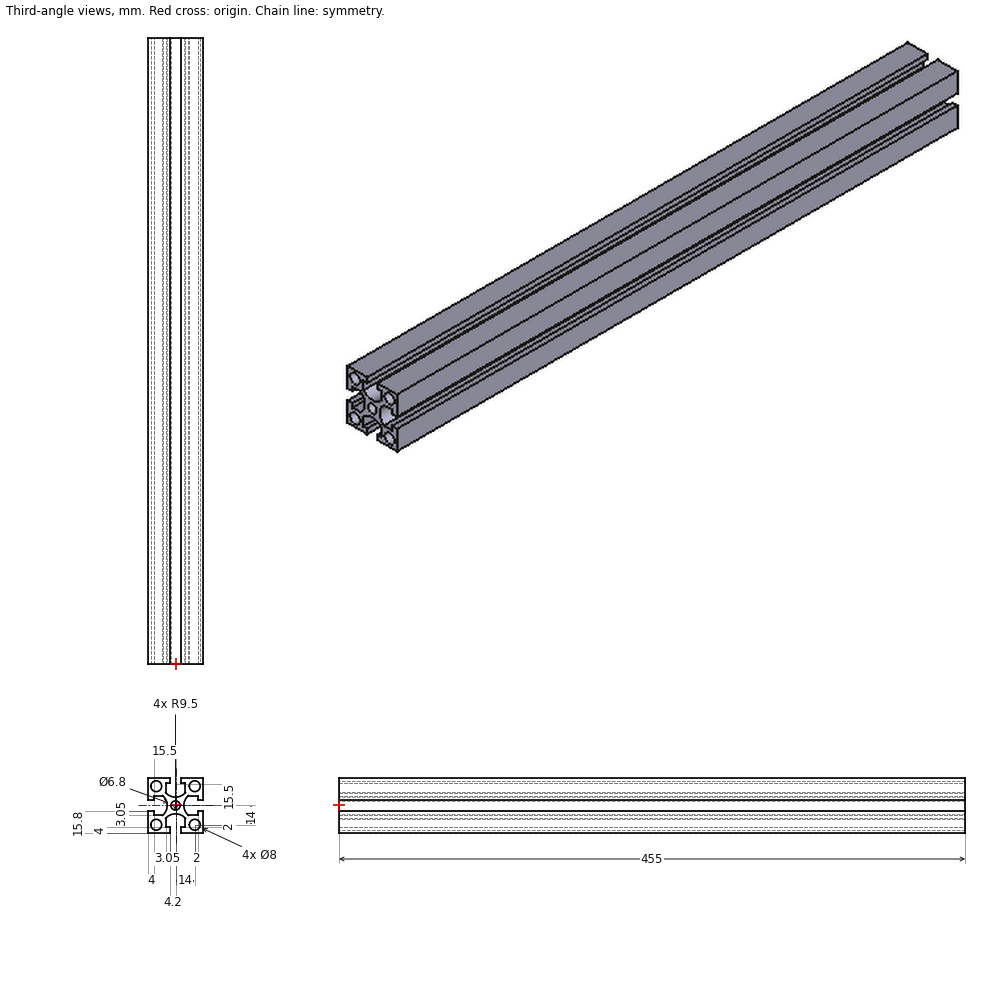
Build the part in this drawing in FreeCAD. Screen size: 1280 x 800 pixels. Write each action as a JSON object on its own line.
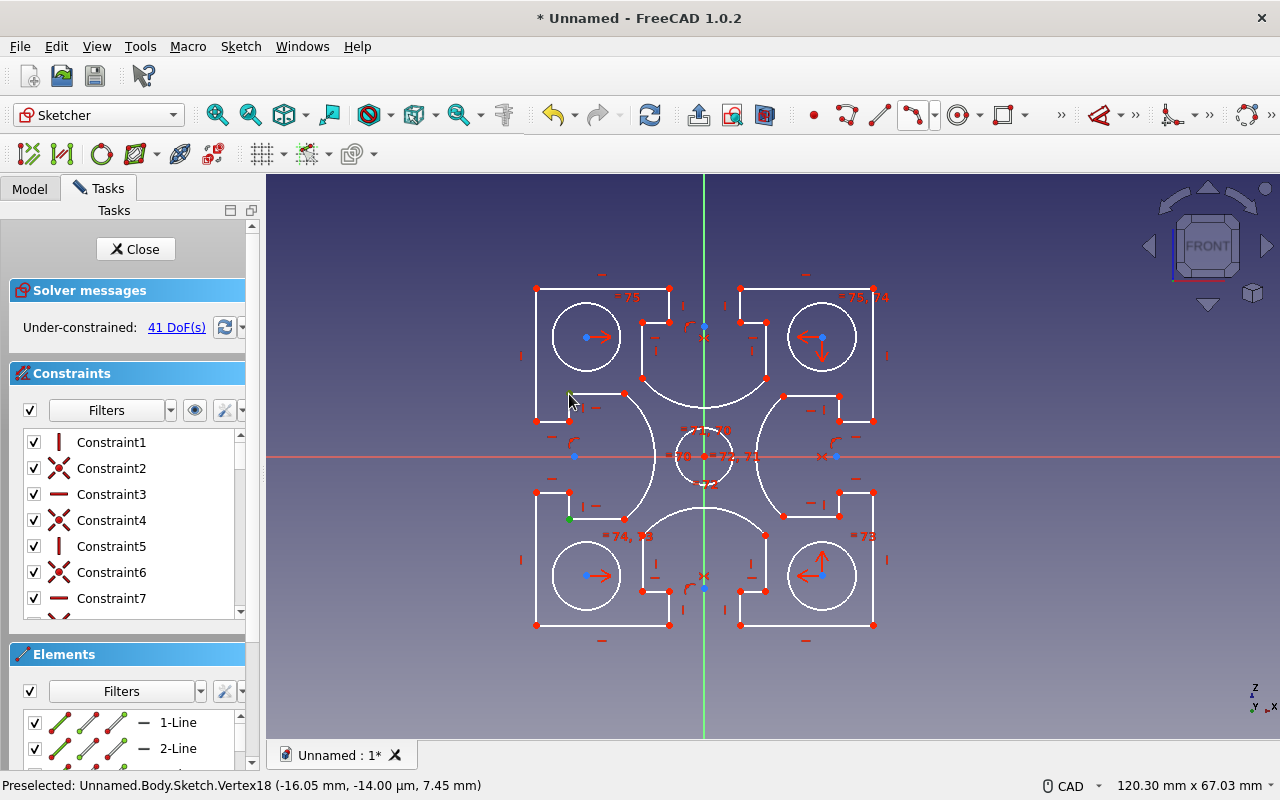
{"action": "left_click", "coordinate": [353, 456]}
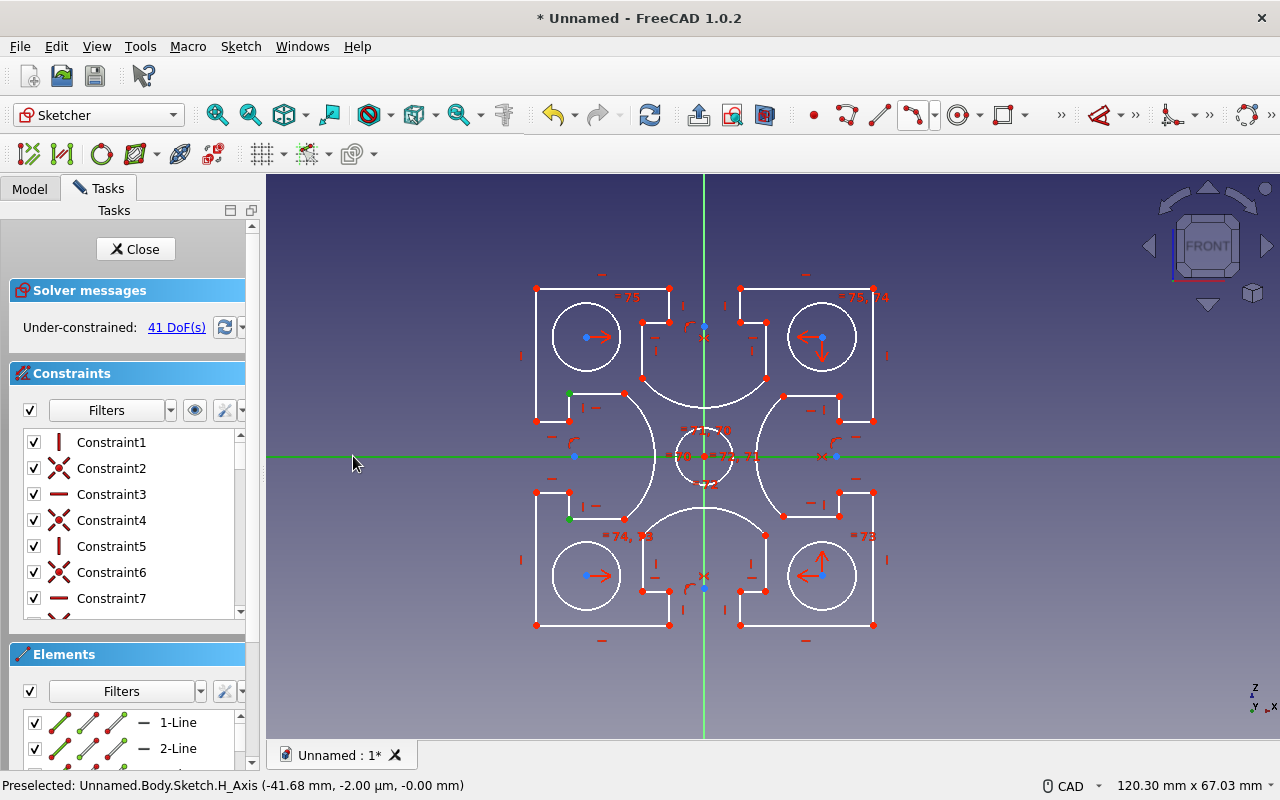
{"action": "key", "text": "s"}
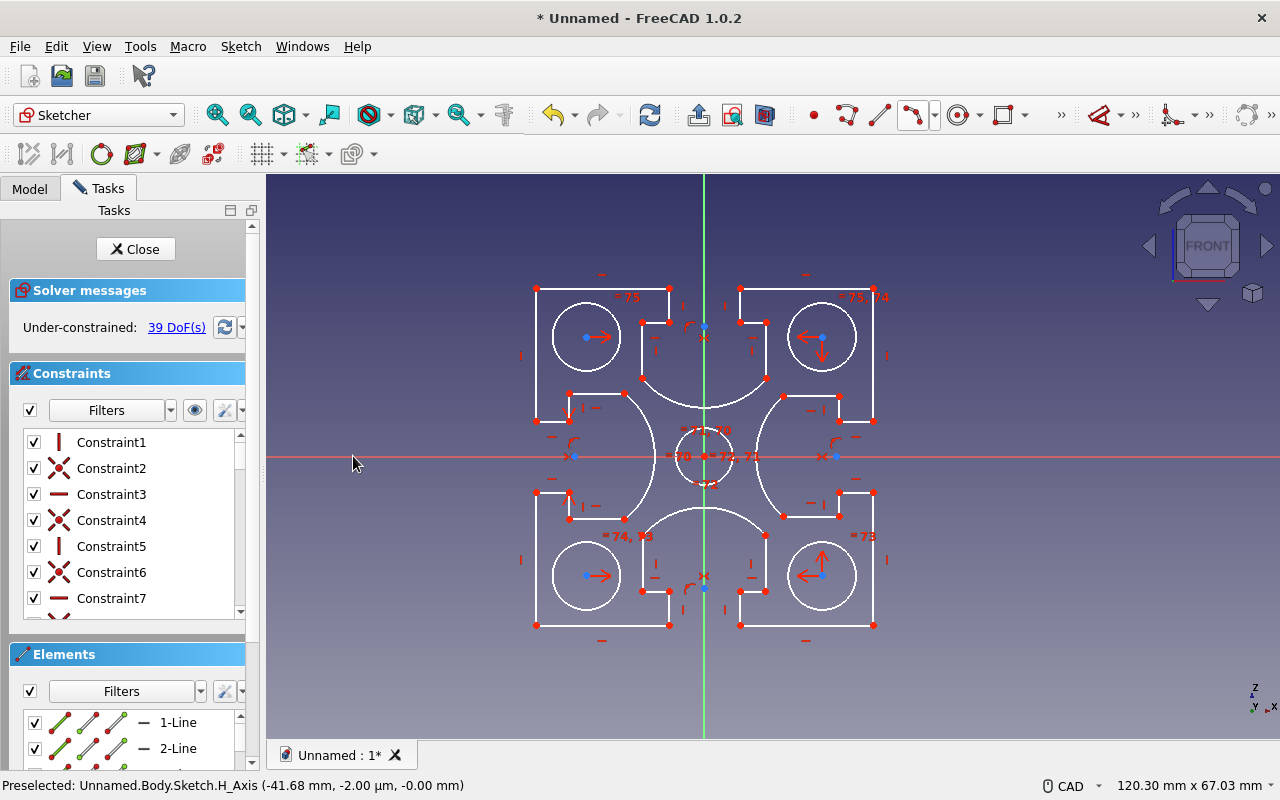
{"action": "left_click", "coordinate": [536, 493]}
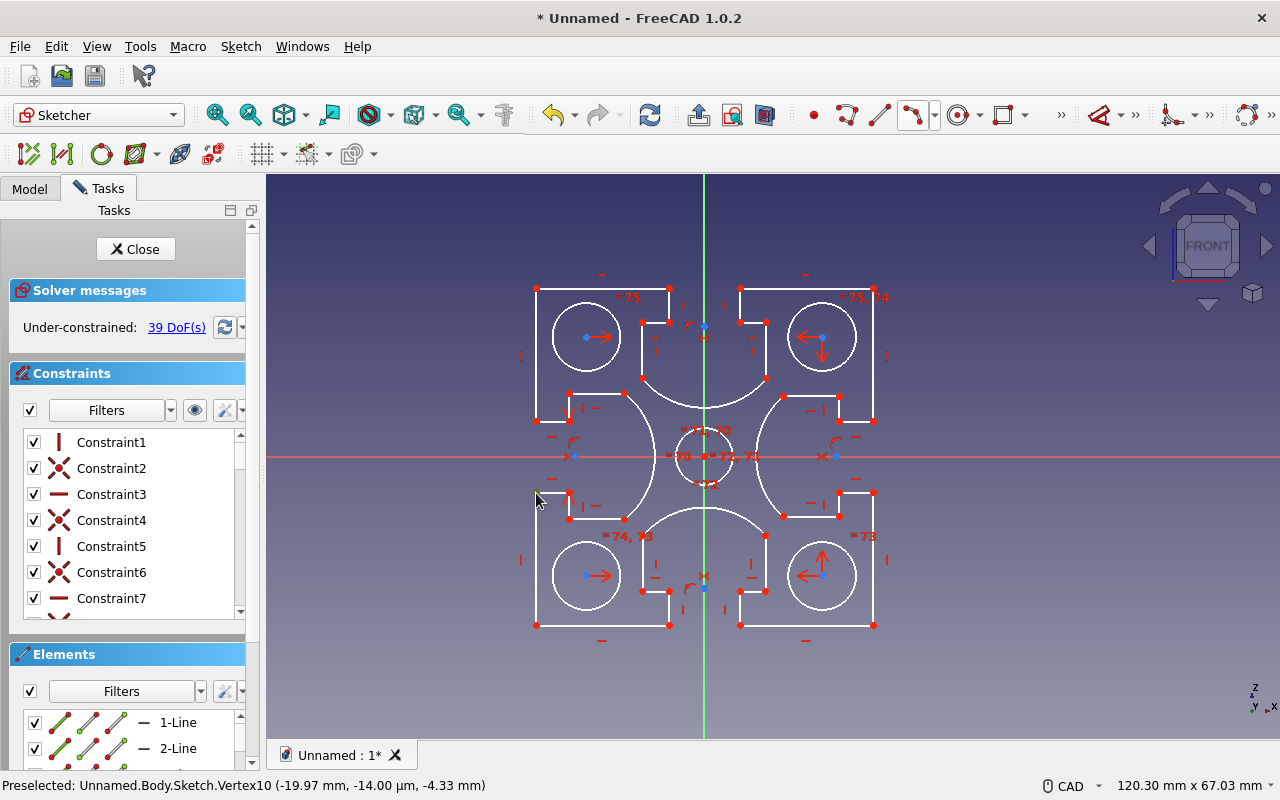
{"action": "left_click", "coordinate": [536, 422]}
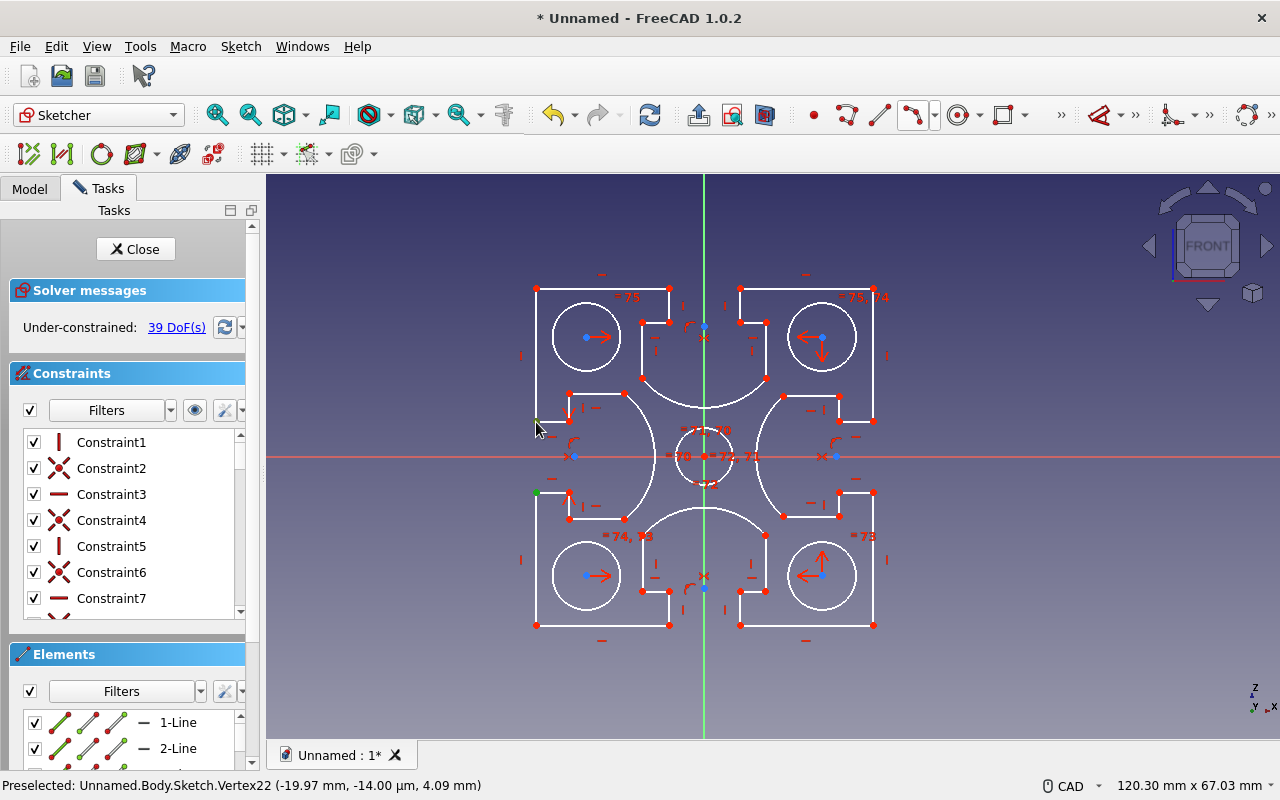
{"action": "left_click", "coordinate": [353, 456]}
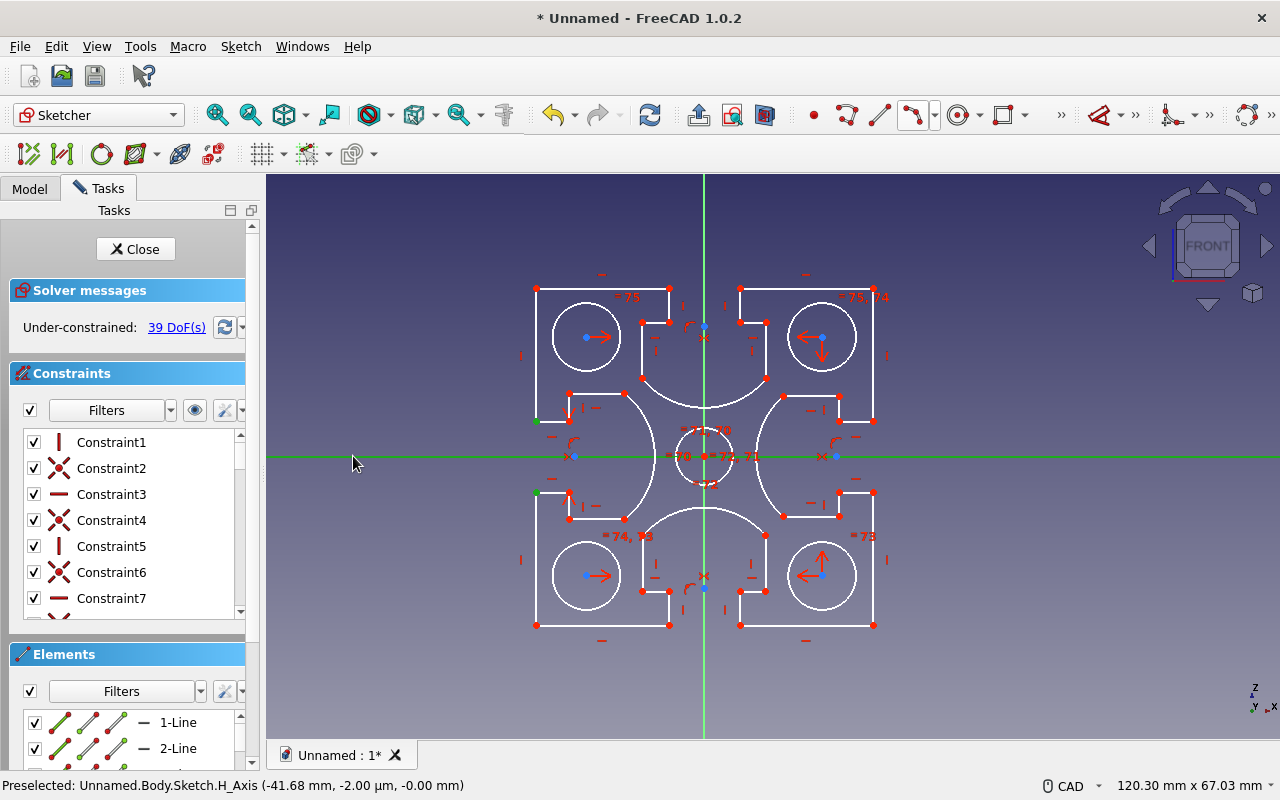
{"action": "key", "text": "s"}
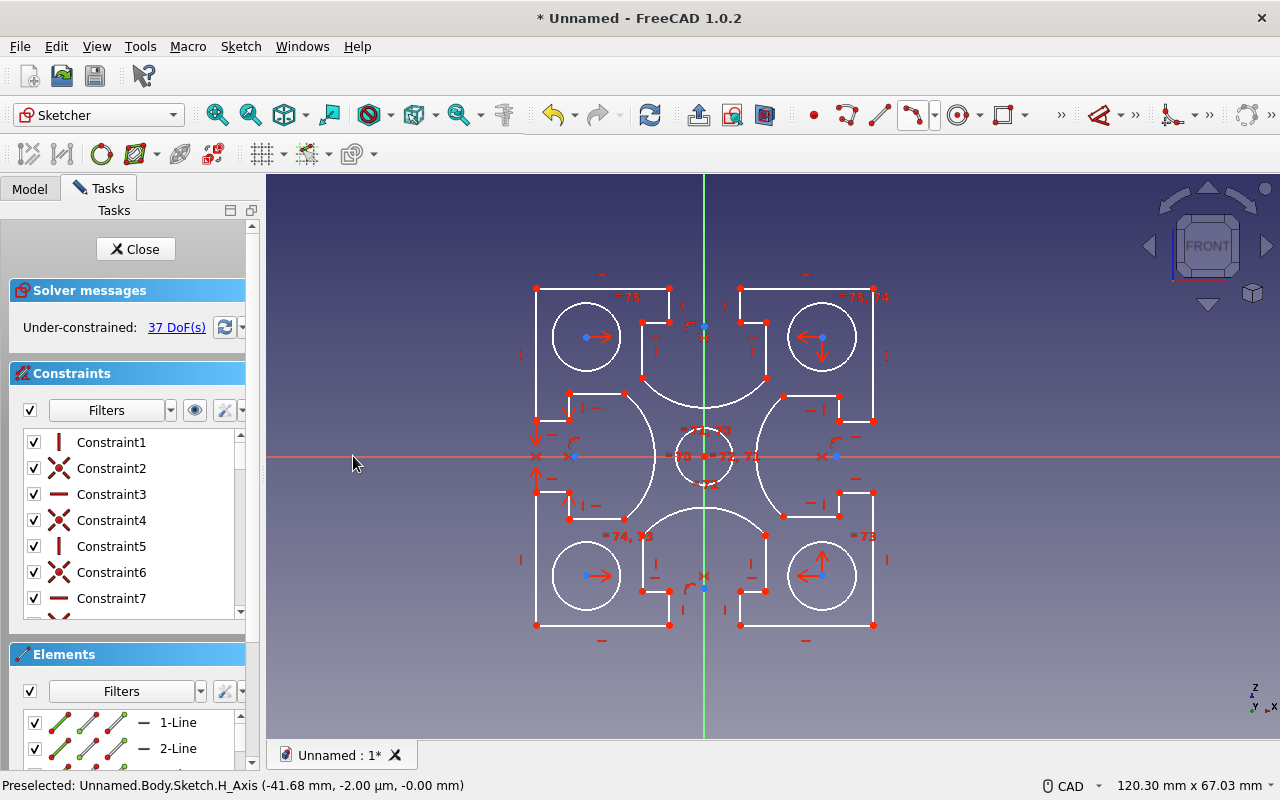
{"action": "left_click", "coordinate": [669, 626]}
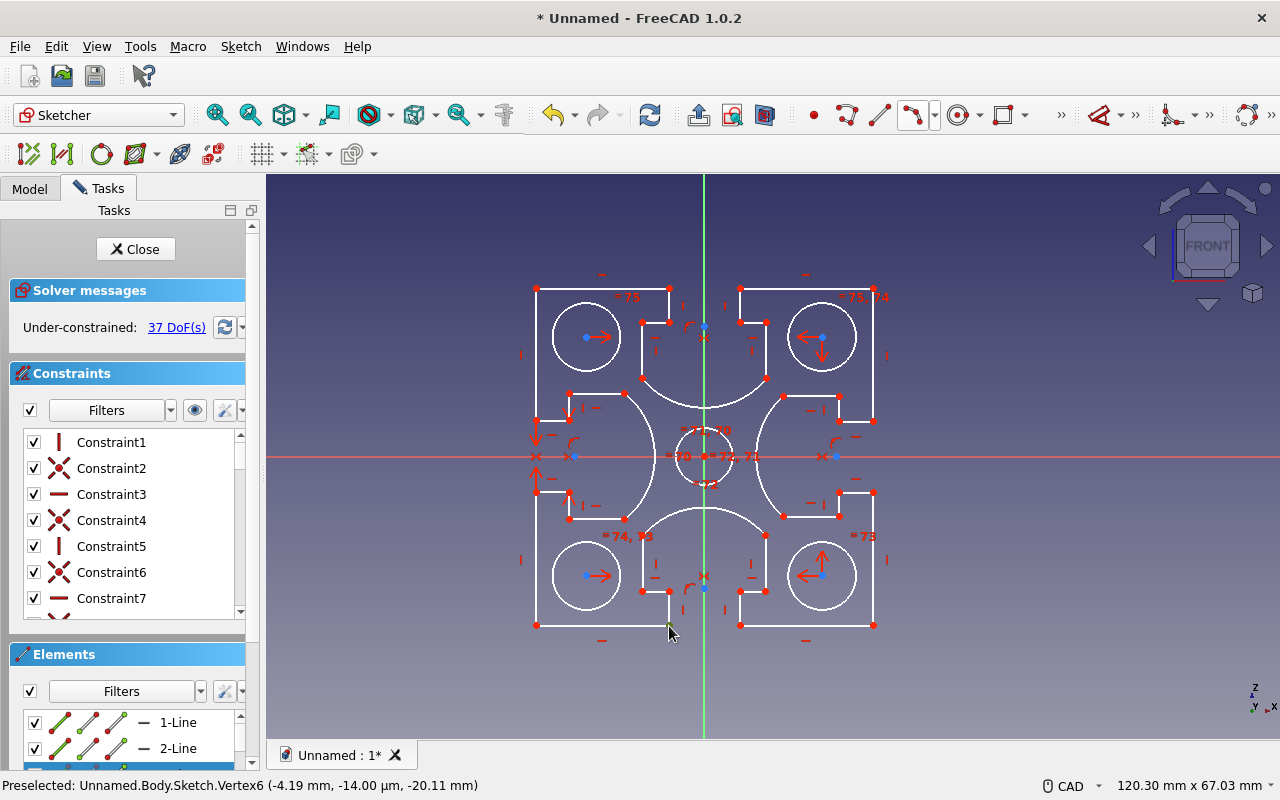
{"action": "left_click", "coordinate": [669, 289]}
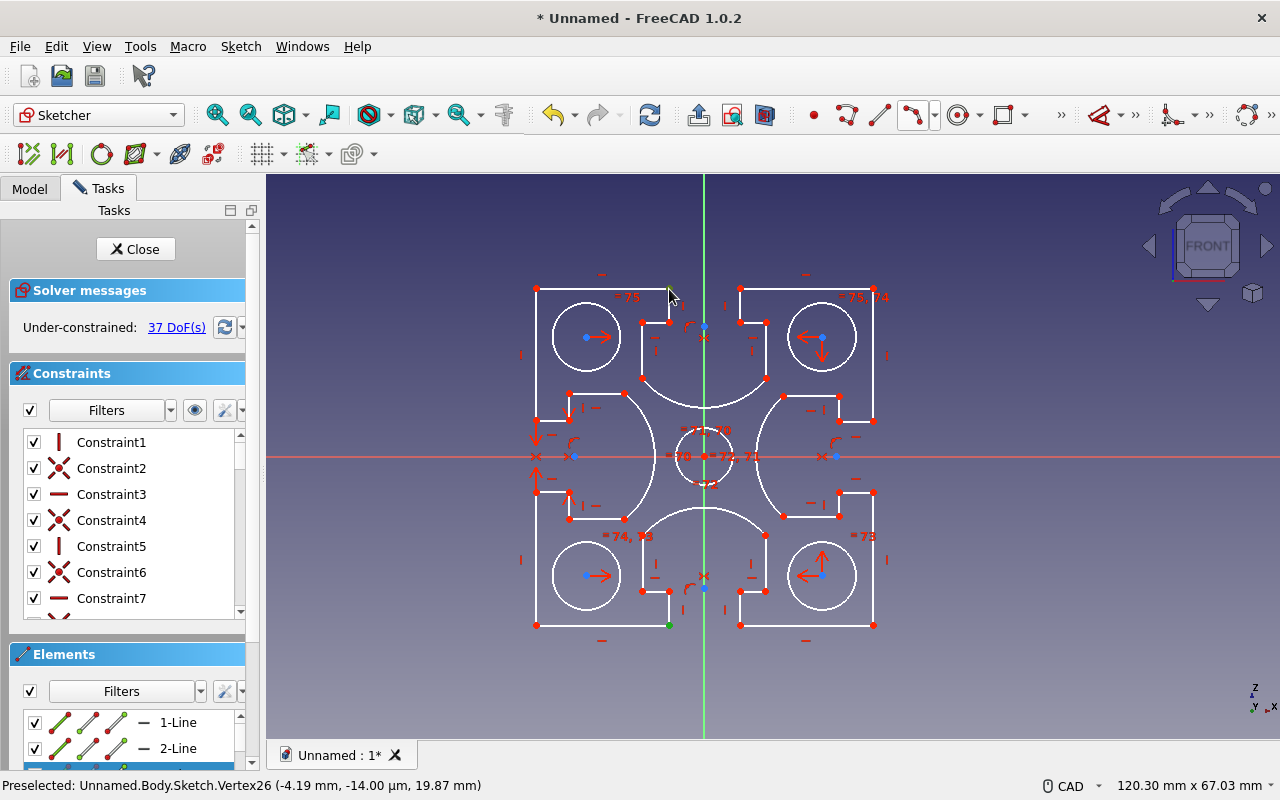
{"action": "left_click", "coordinate": [353, 456]}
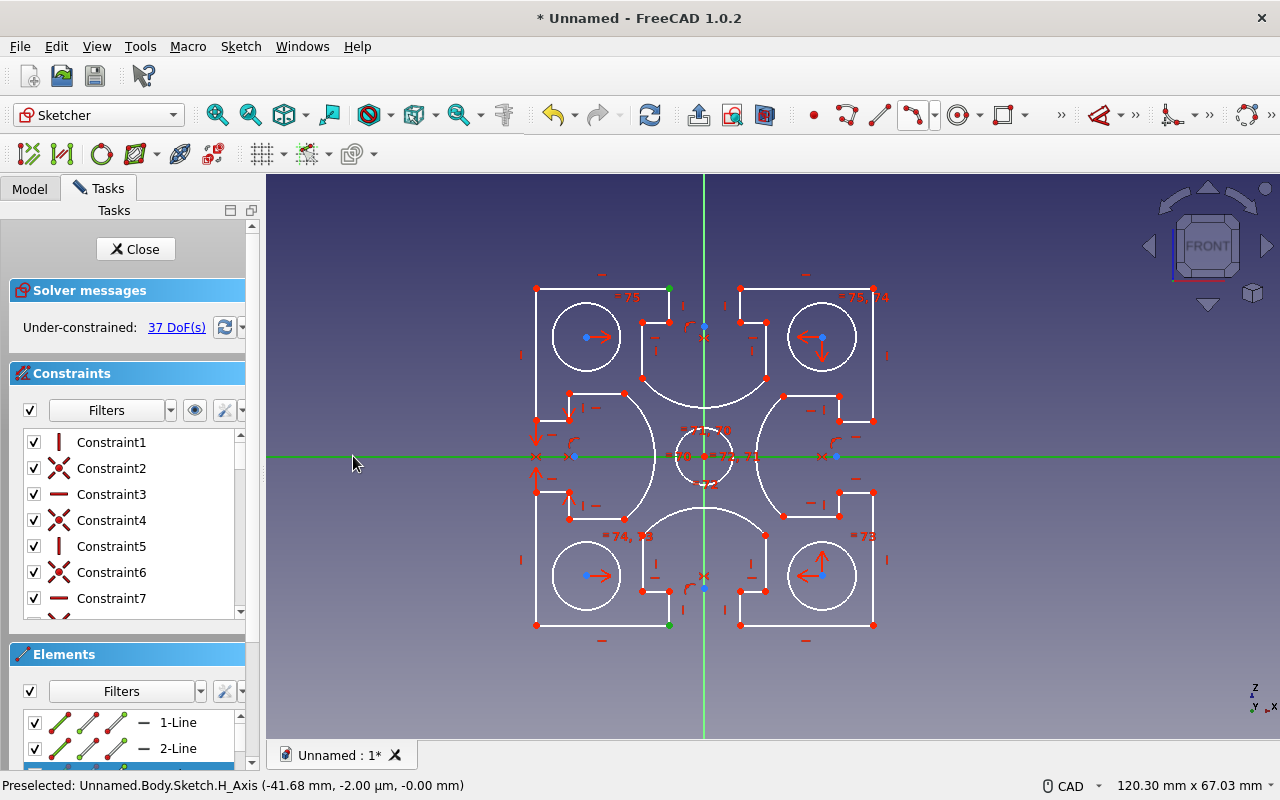
{"action": "key", "text": "s"}